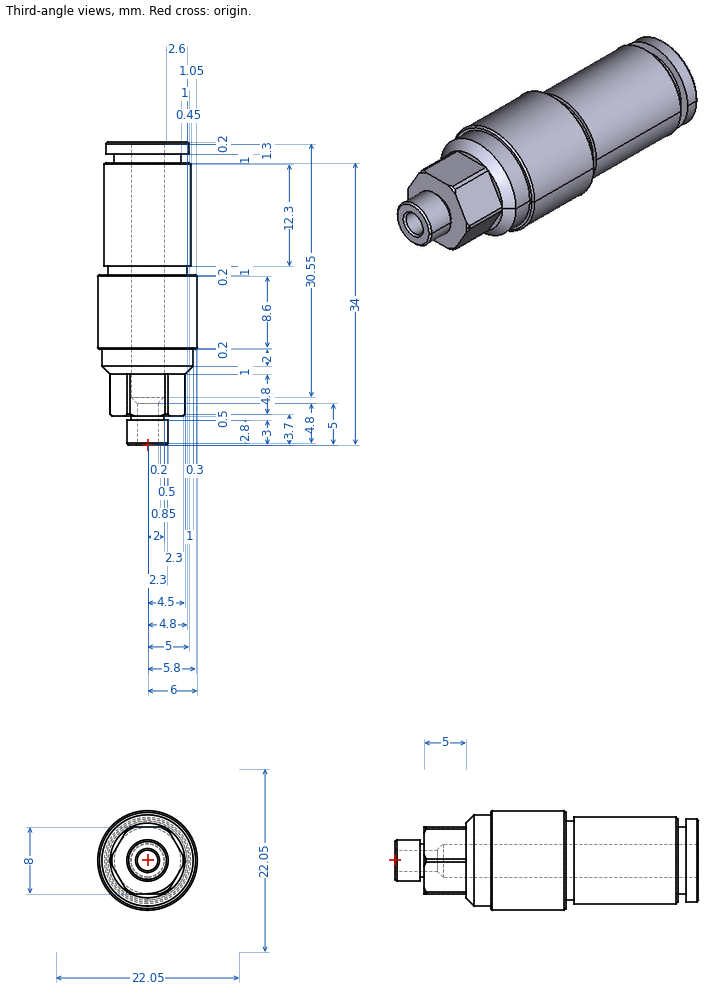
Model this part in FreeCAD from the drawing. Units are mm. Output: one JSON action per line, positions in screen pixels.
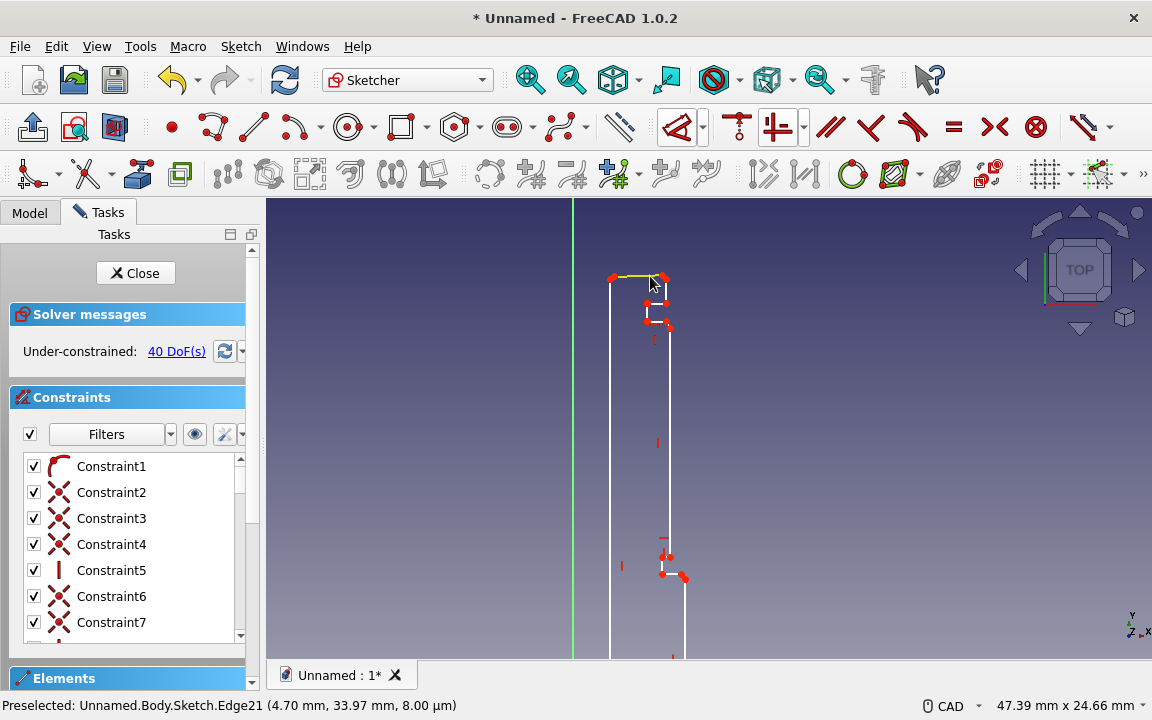
{"action": "left_click", "coordinate": [648, 276]}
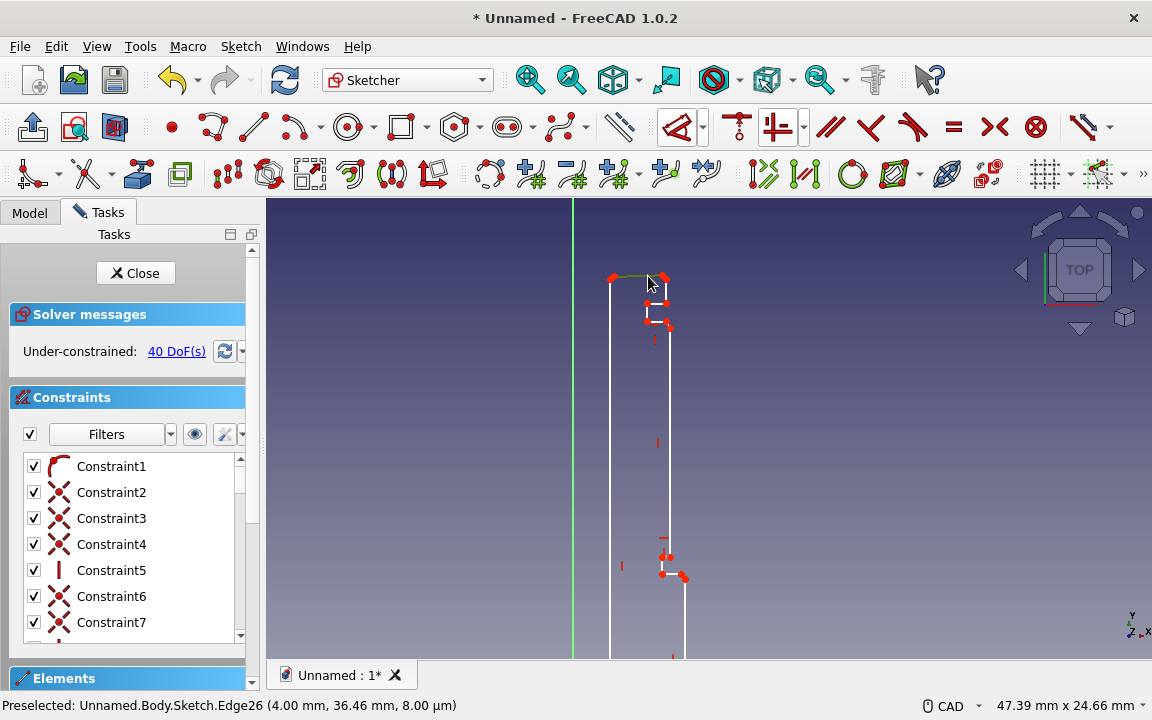
{"action": "key", "text": "h"}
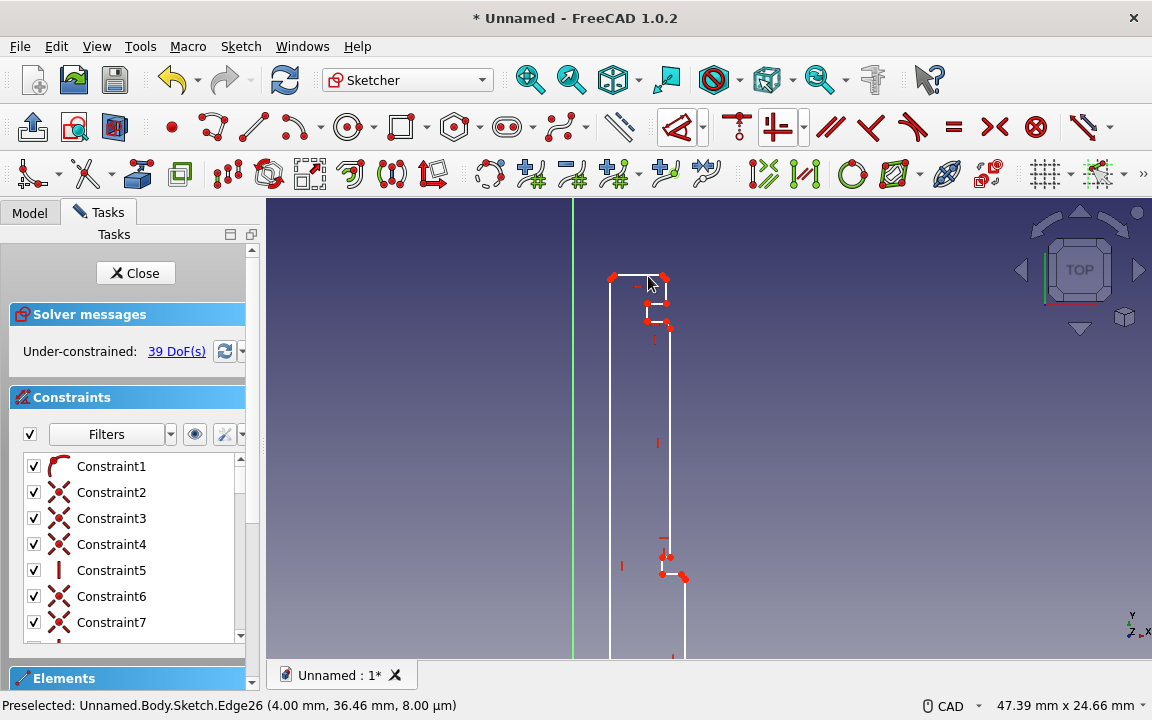
{"action": "scroll", "coordinate": [650, 275], "scroll_direction": "down", "scroll_amount": 4}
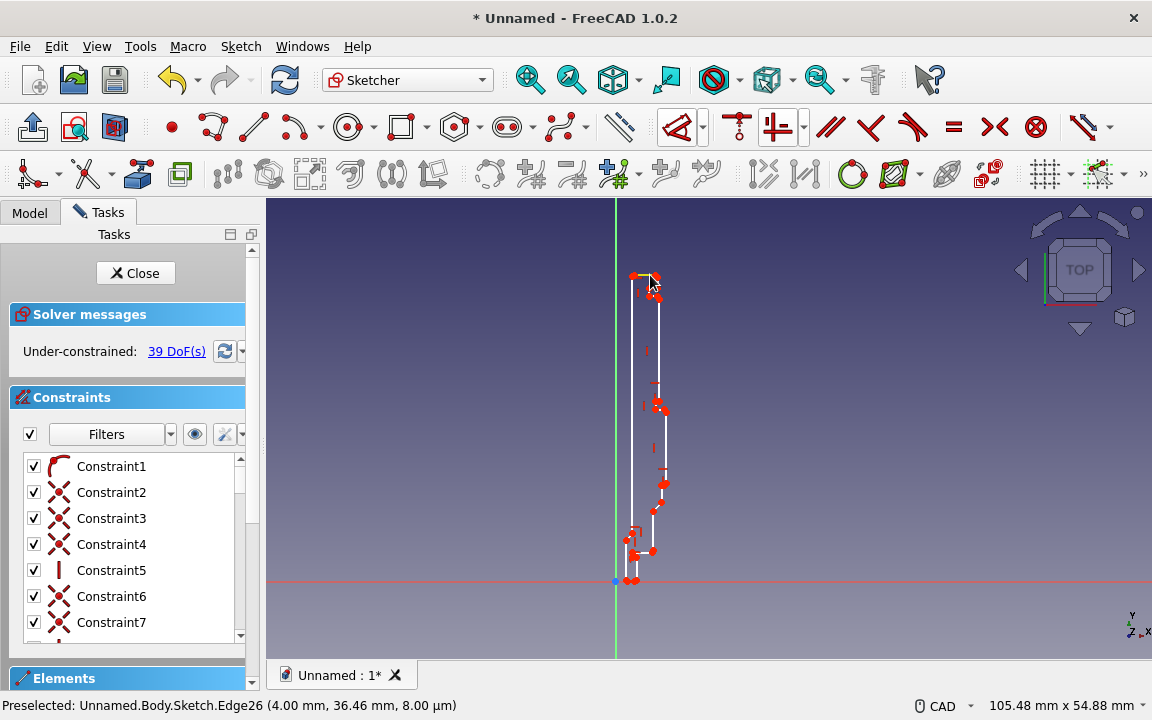
{"action": "scroll", "coordinate": [662, 497], "scroll_direction": "up", "scroll_amount": 6}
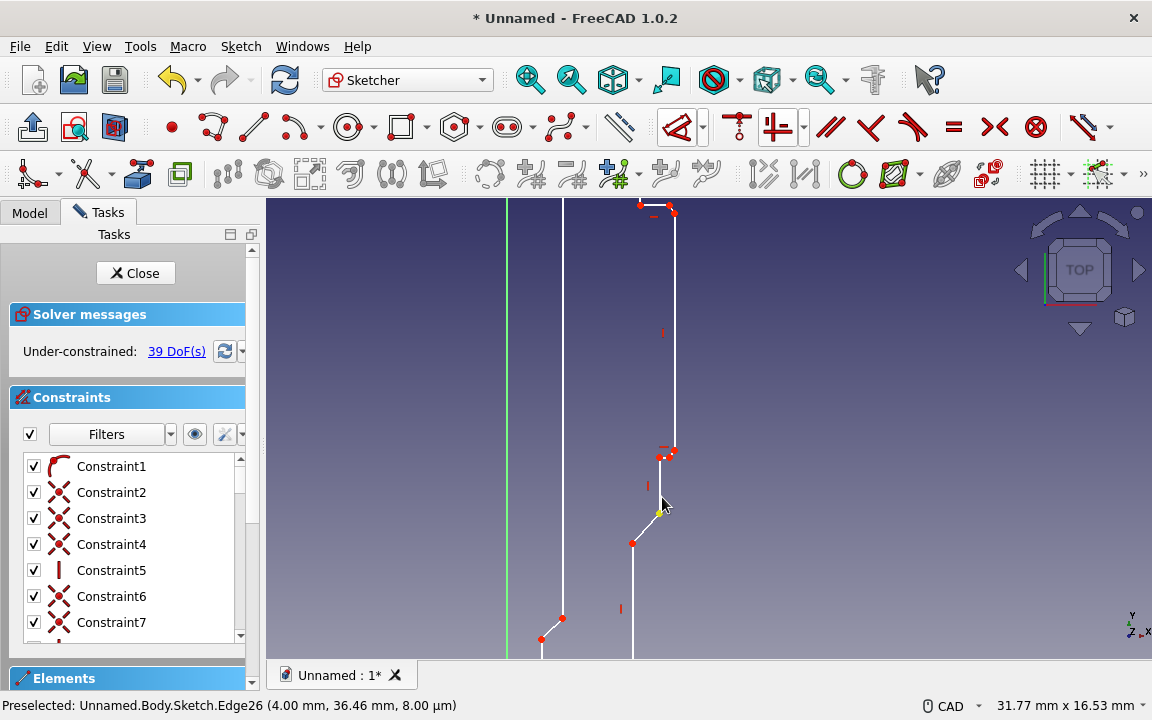
{"action": "left_click", "coordinate": [660, 497]}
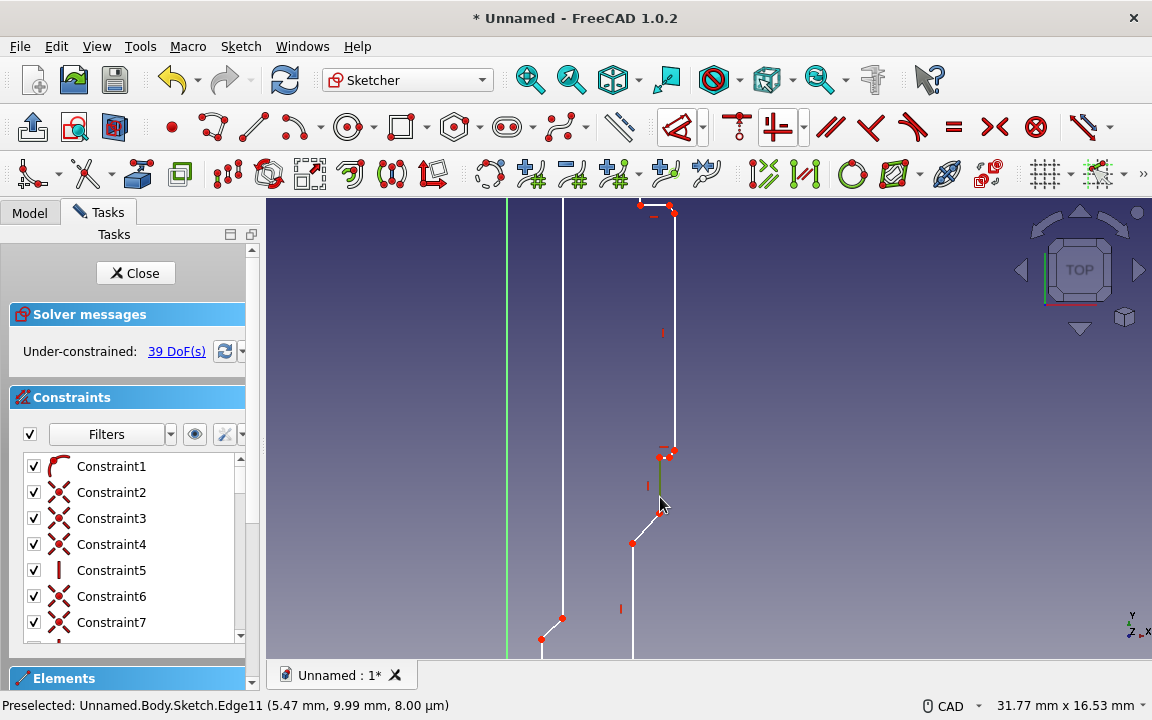
{"action": "left_click", "coordinate": [702, 128]}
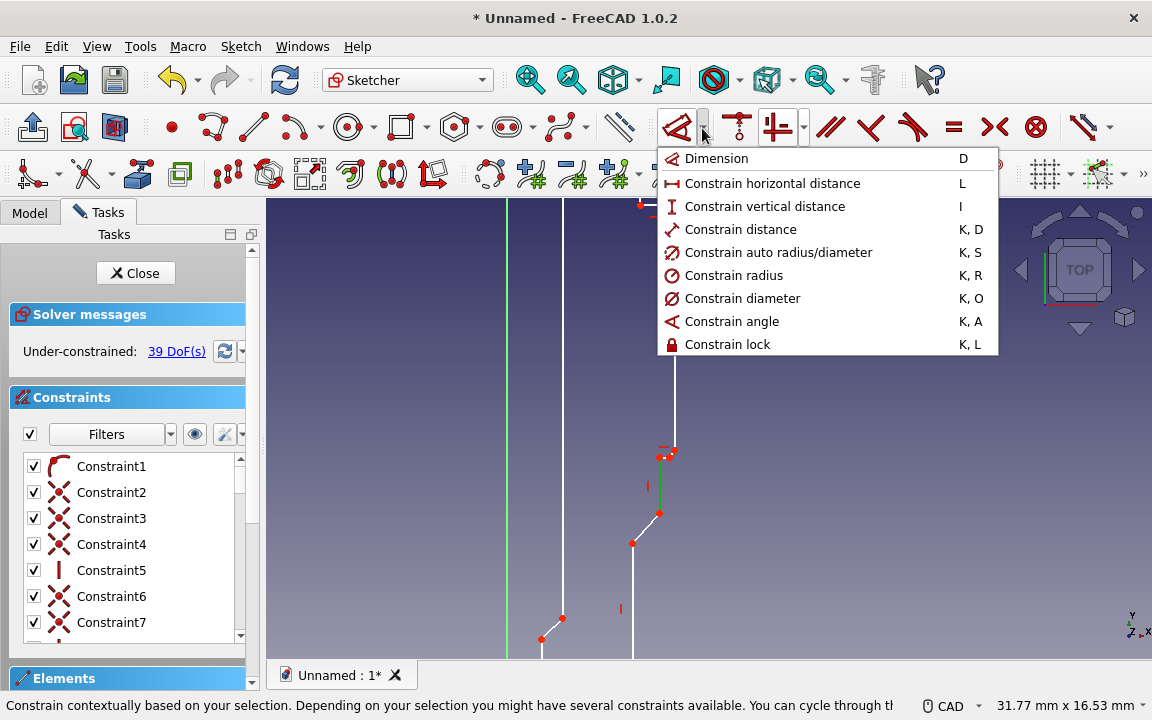
{"action": "left_click", "coordinate": [828, 206]}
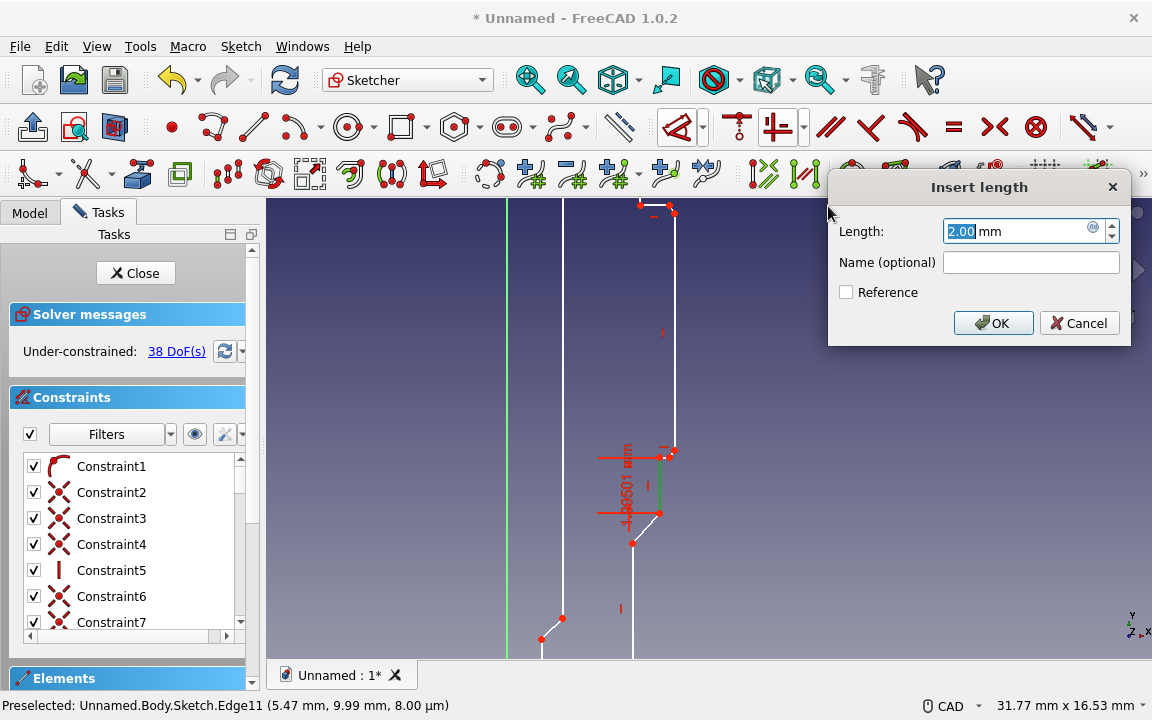
{"action": "type", "text": "2"}
{"action": "key", "text": "Return"}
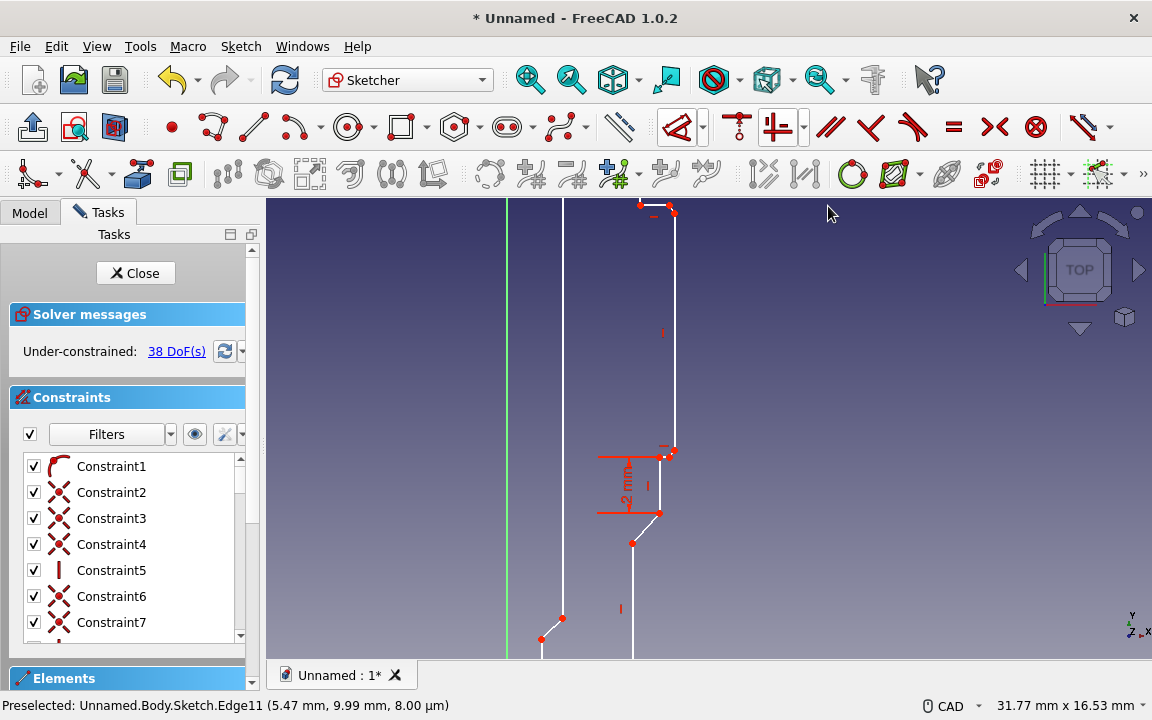
{"action": "scroll", "coordinate": [662, 498], "scroll_direction": "down", "scroll_amount": 6}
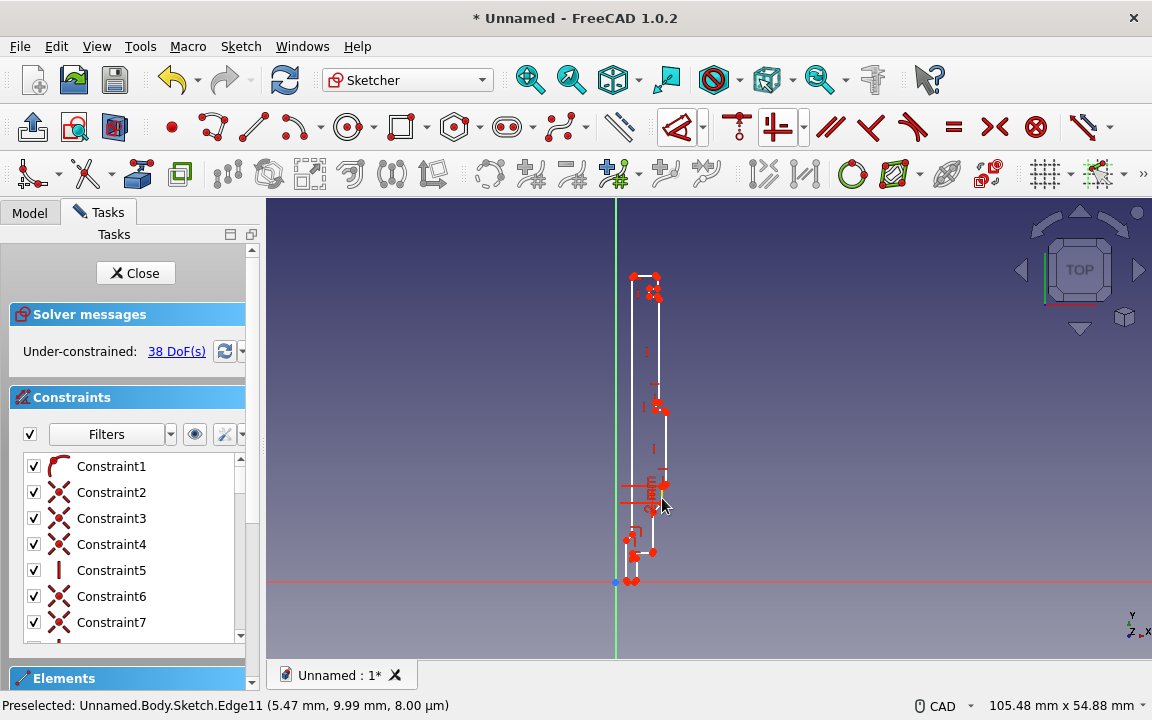
{"action": "scroll", "coordinate": [656, 407], "scroll_direction": "up", "scroll_amount": 8}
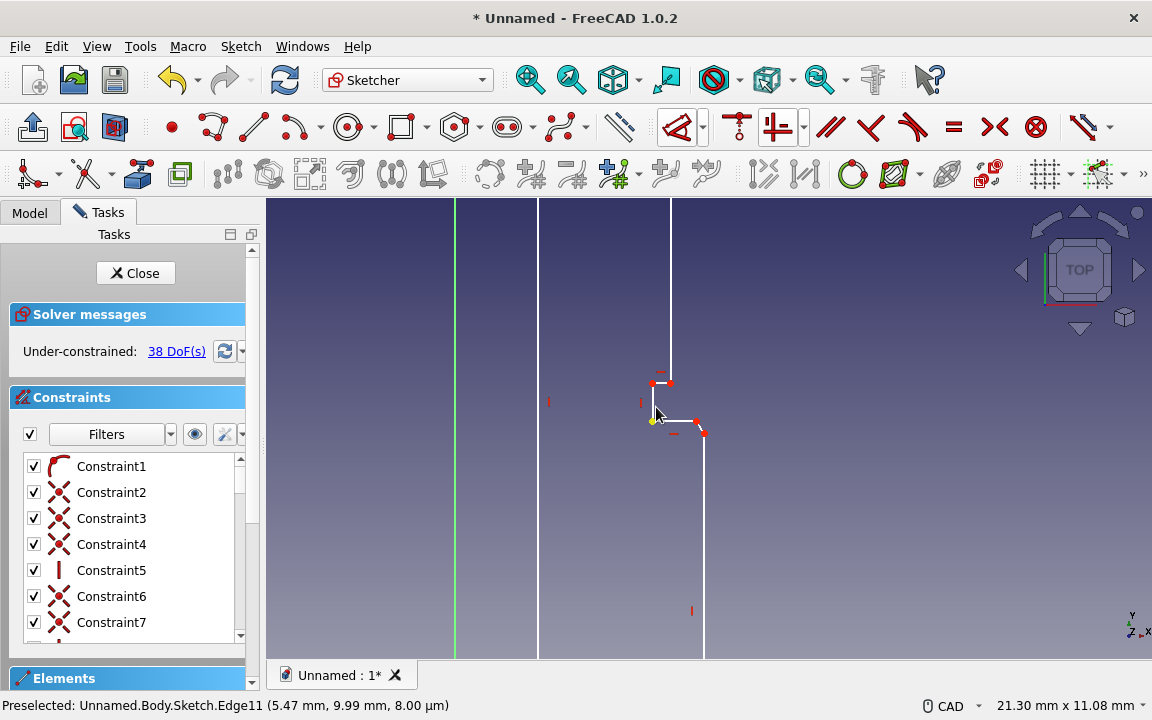
{"action": "left_click", "coordinate": [653, 406]}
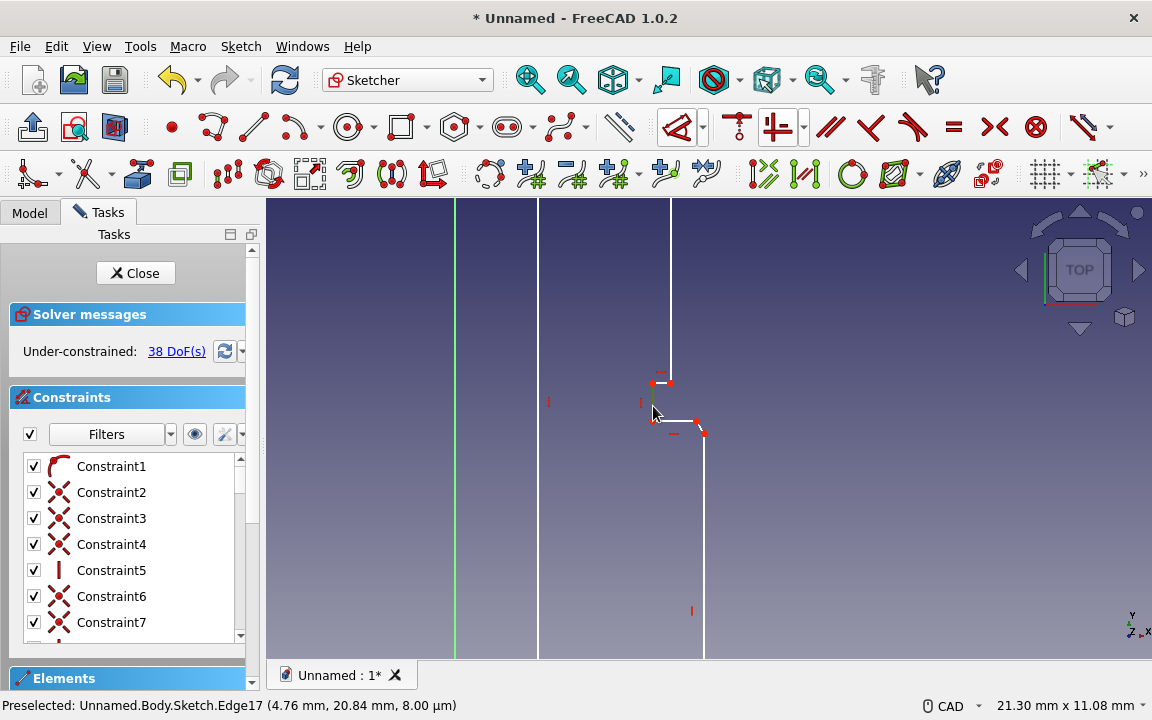
{"action": "left_click", "coordinate": [702, 128]}